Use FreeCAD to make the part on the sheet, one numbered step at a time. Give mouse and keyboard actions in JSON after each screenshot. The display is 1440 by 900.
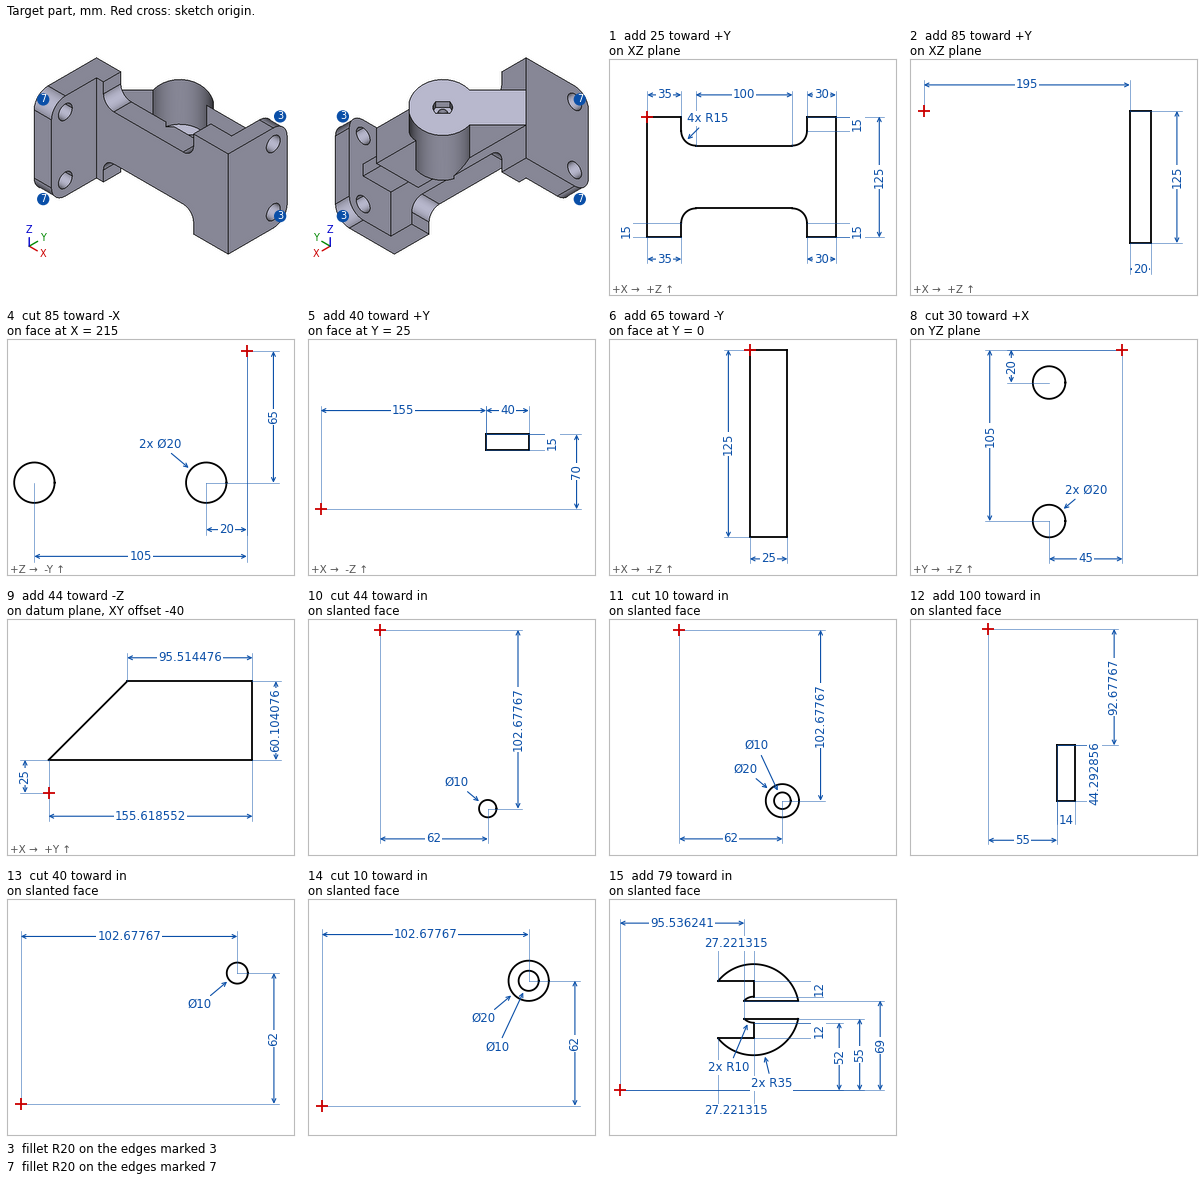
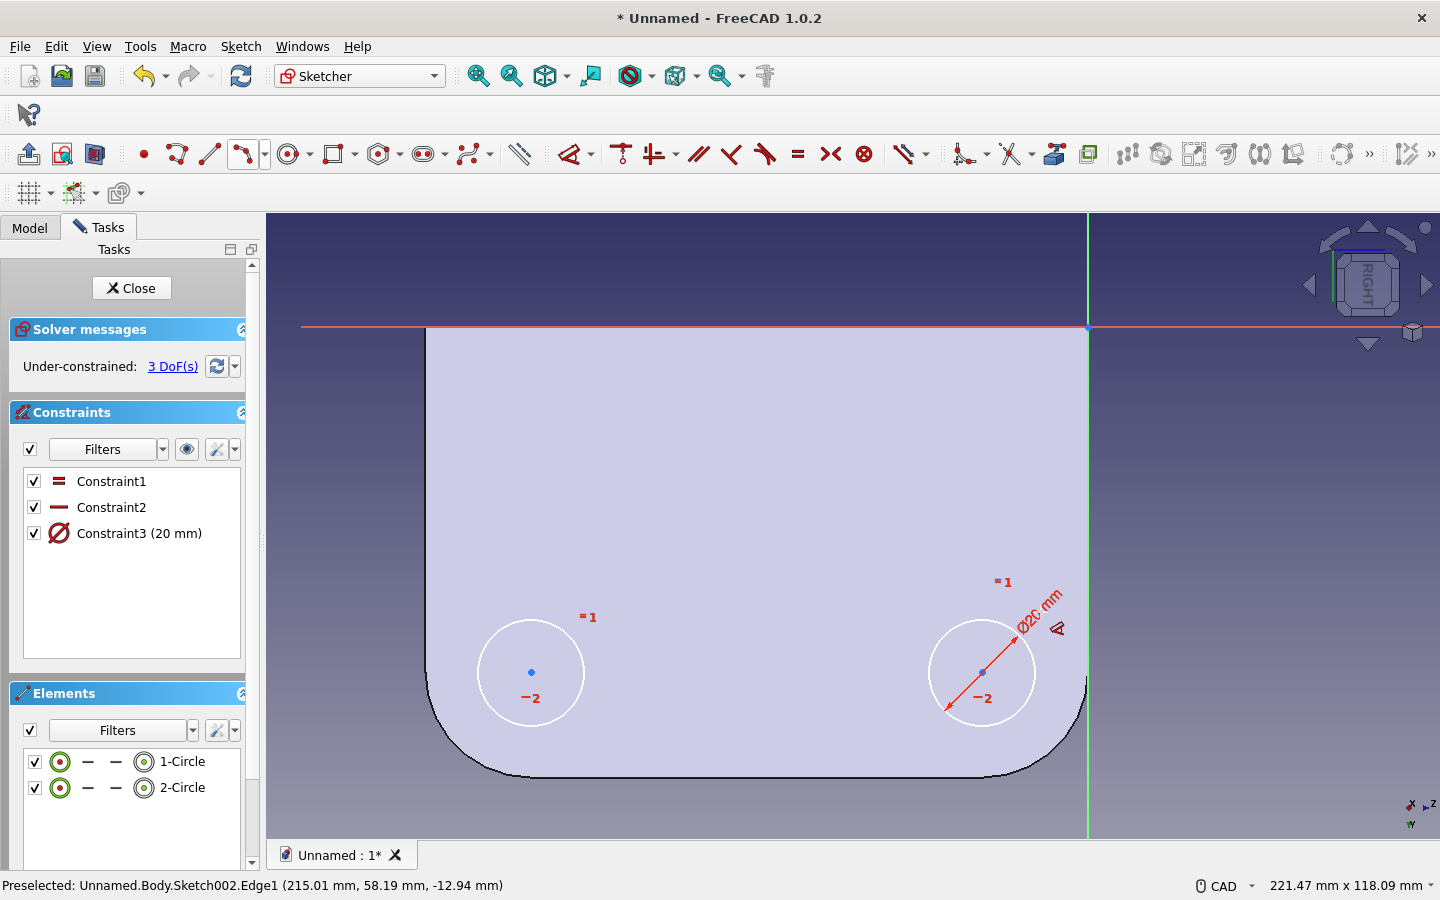
{"action": "left_click", "coordinate": [982, 673]}
{"action": "left_click", "coordinate": [1035, 293]}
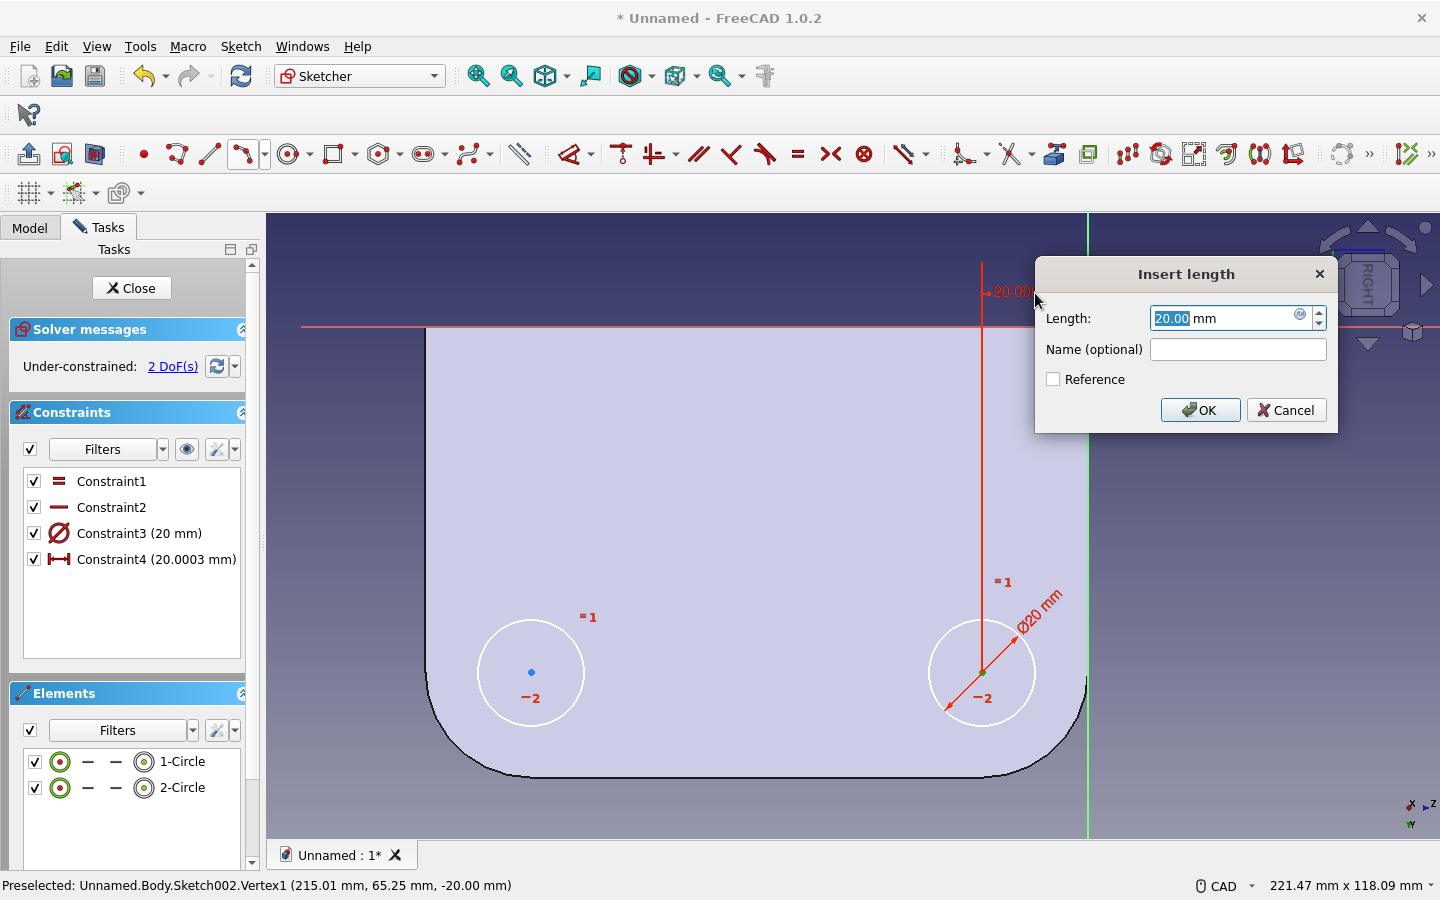
{"action": "type", "text": "20"}
{"action": "key", "text": "Return"}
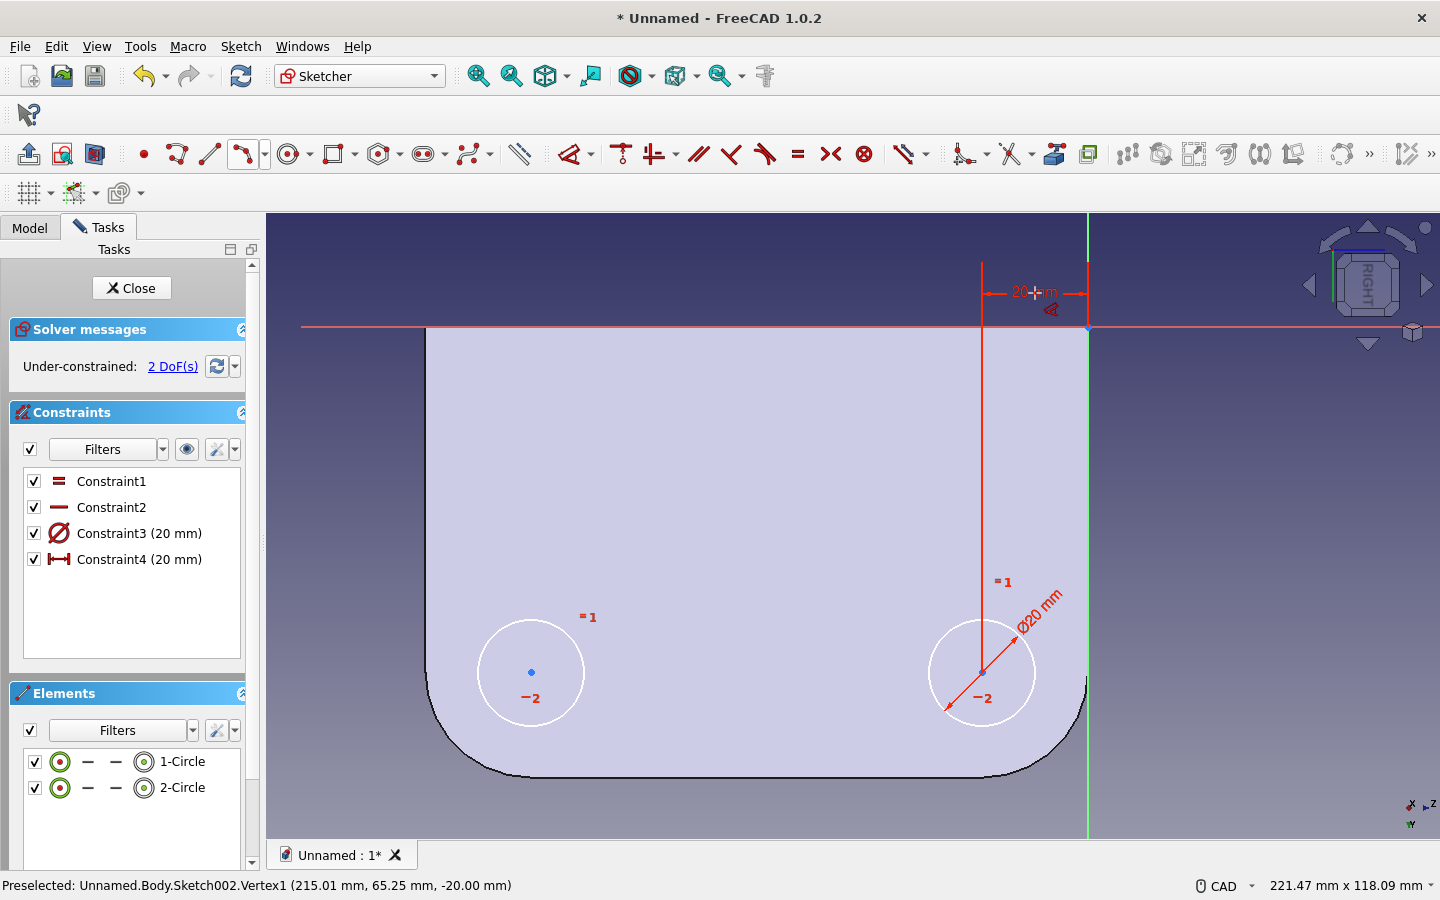
{"action": "left_click", "coordinate": [982, 673]}
{"action": "left_click", "coordinate": [1122, 500]}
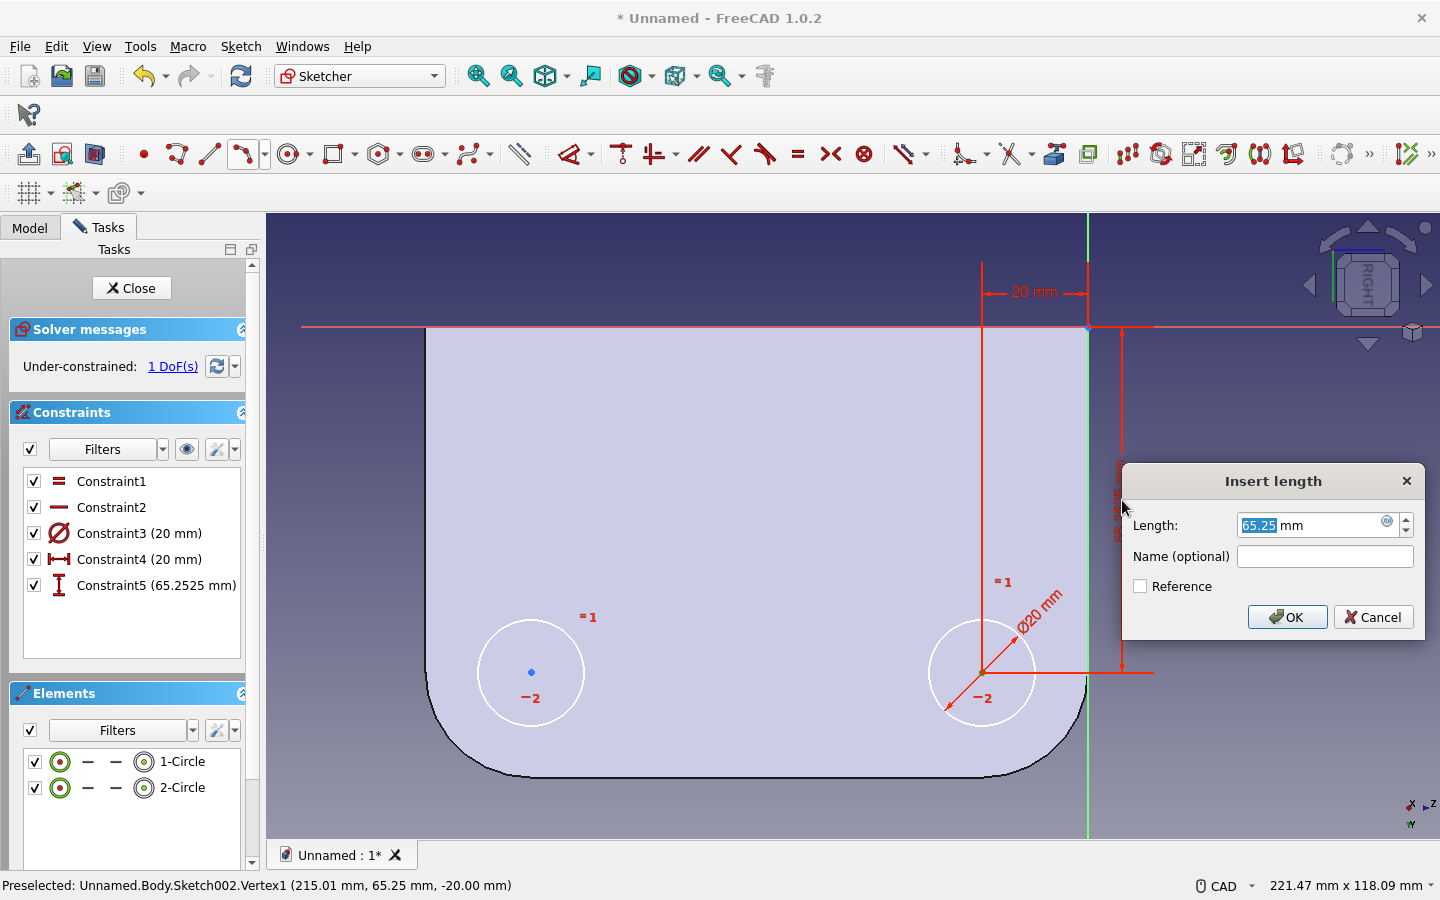
{"action": "type", "text": "65"}
{"action": "key", "text": "Return"}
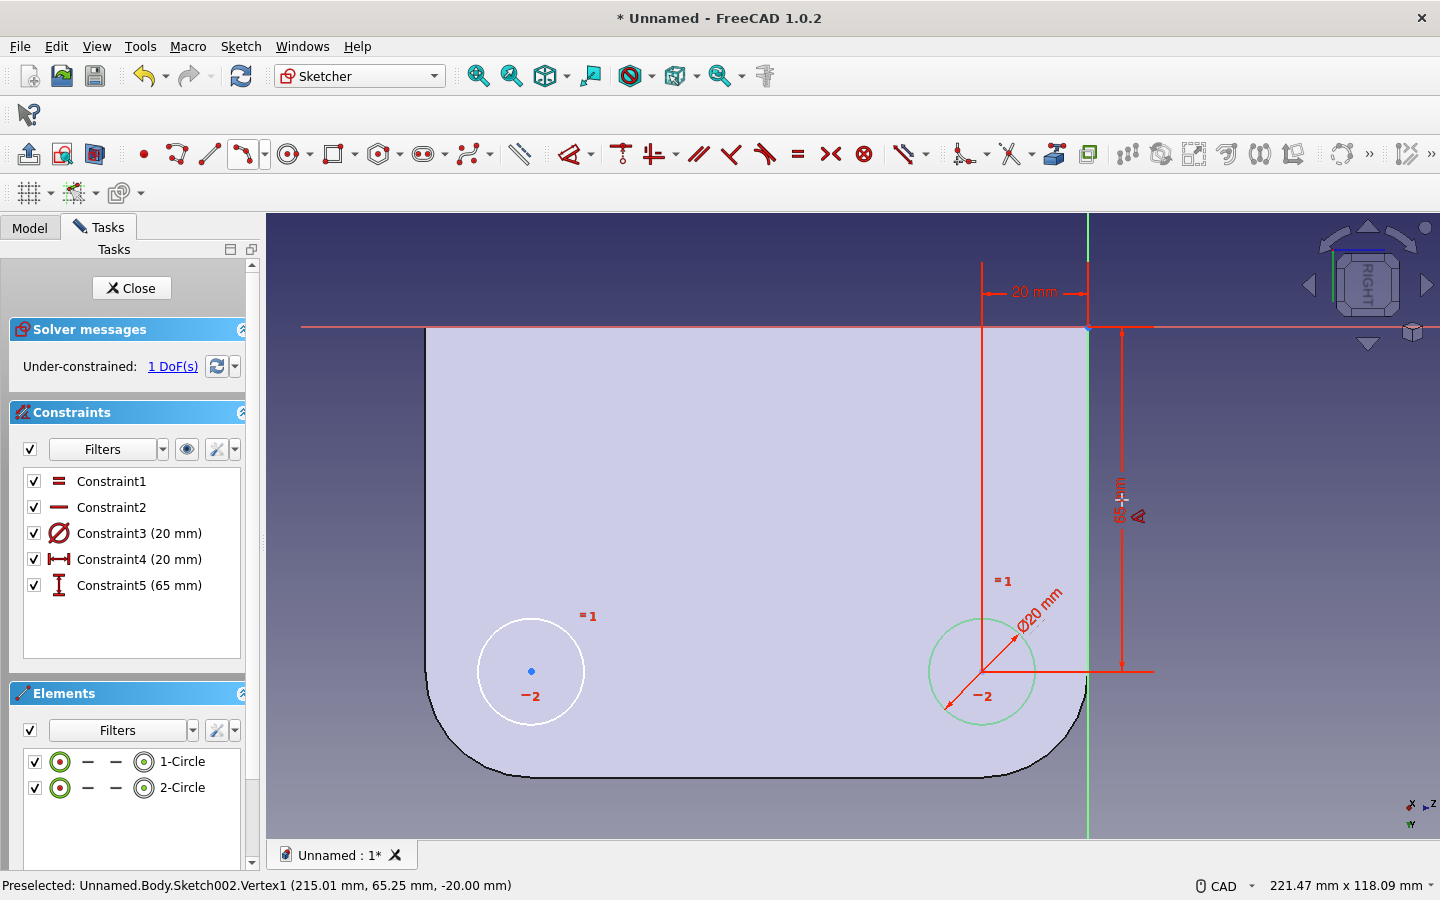
{"action": "left_click", "coordinate": [531, 672]}
{"action": "left_click", "coordinate": [810, 293]}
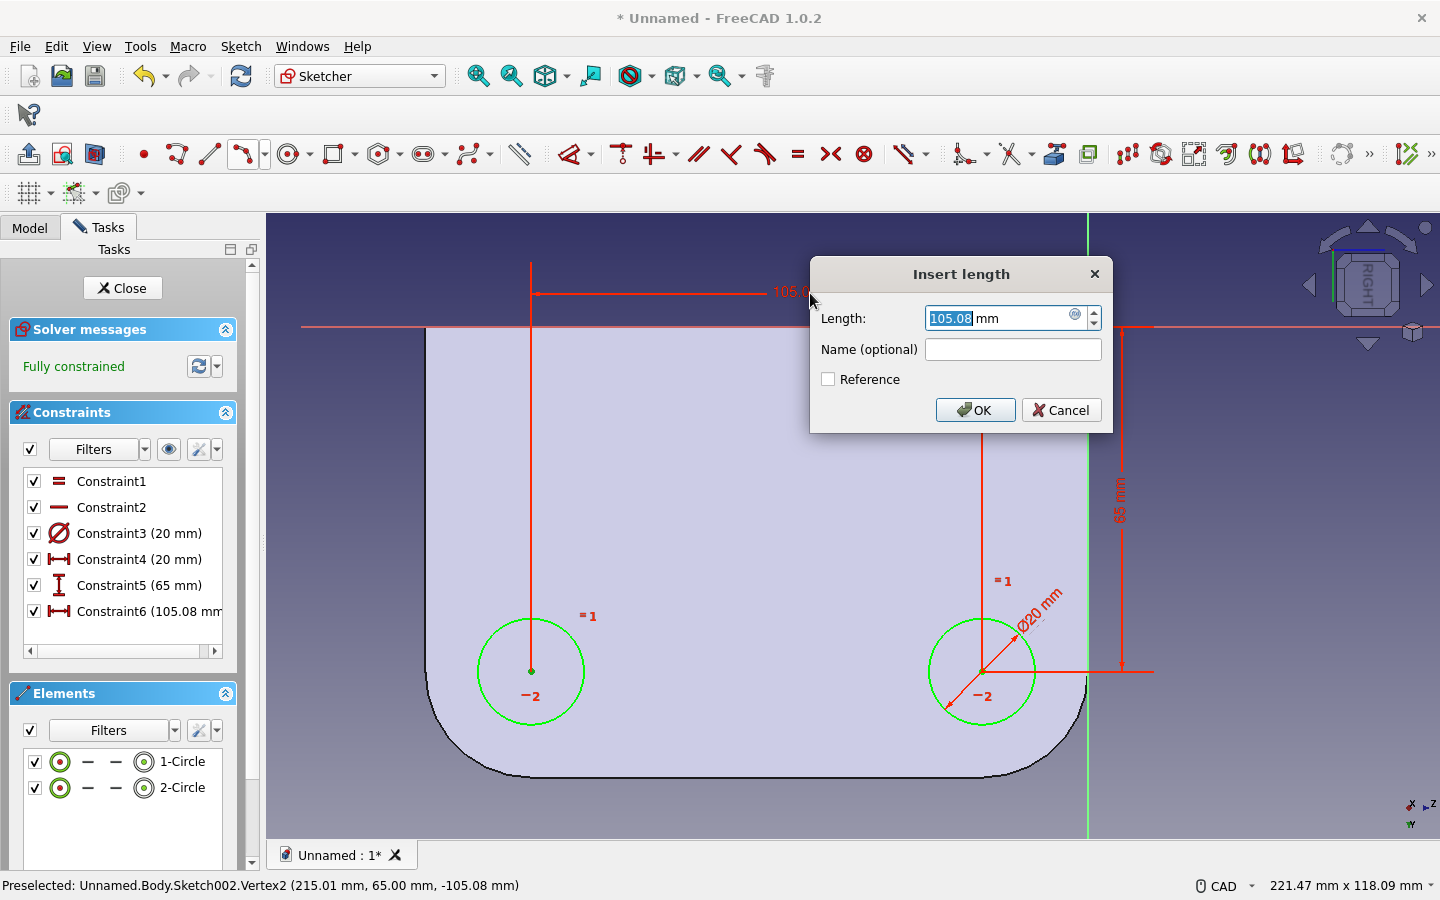
{"action": "type", "text": "105"}
{"action": "key", "text": "Return"}
{"action": "key", "text": "Escape"}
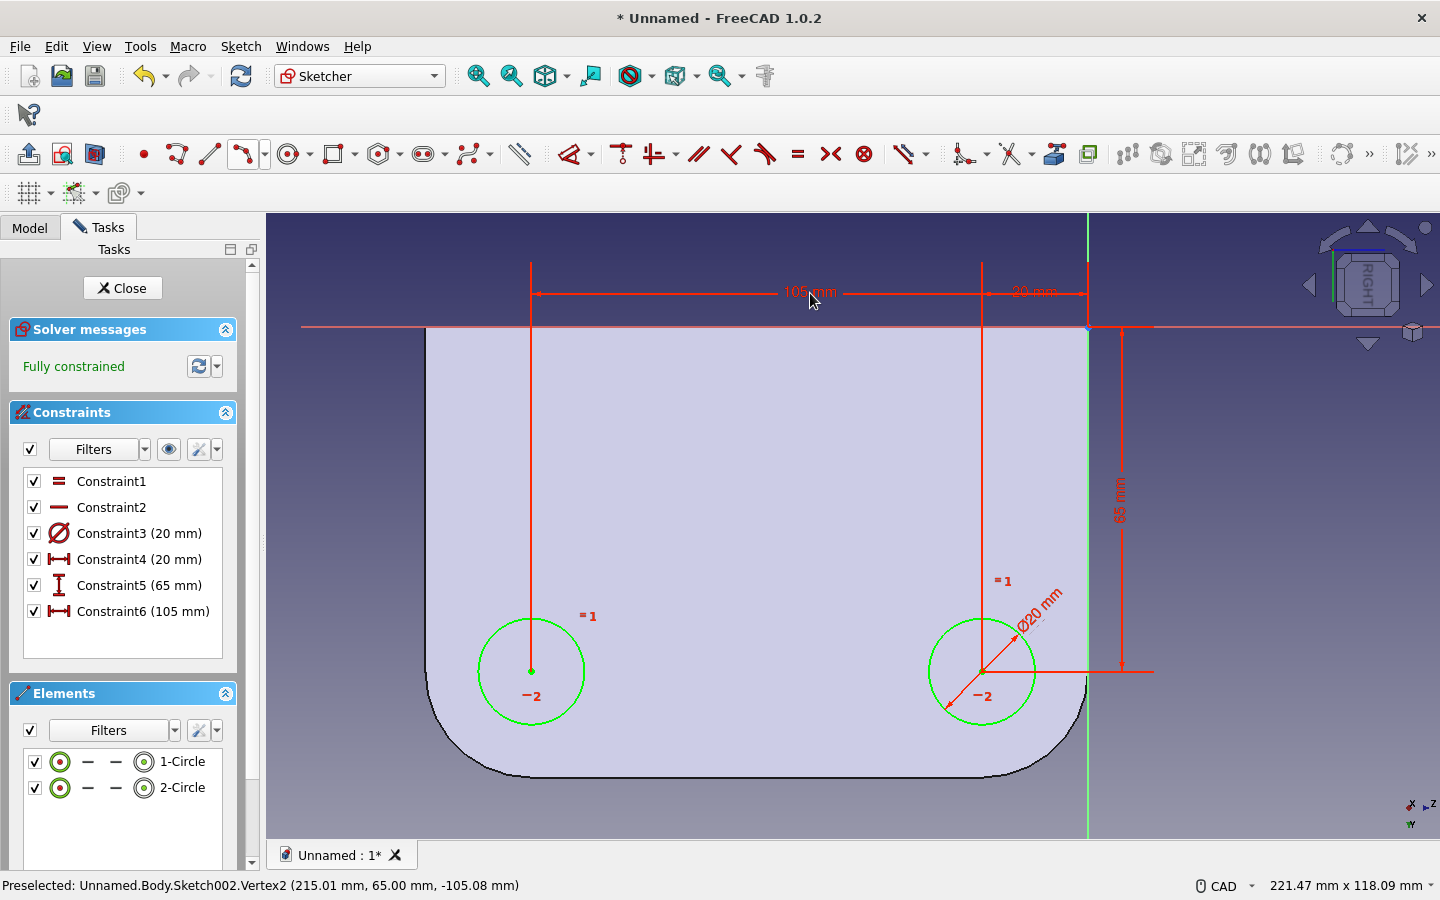
{"action": "left_click", "coordinate": [123, 288]}